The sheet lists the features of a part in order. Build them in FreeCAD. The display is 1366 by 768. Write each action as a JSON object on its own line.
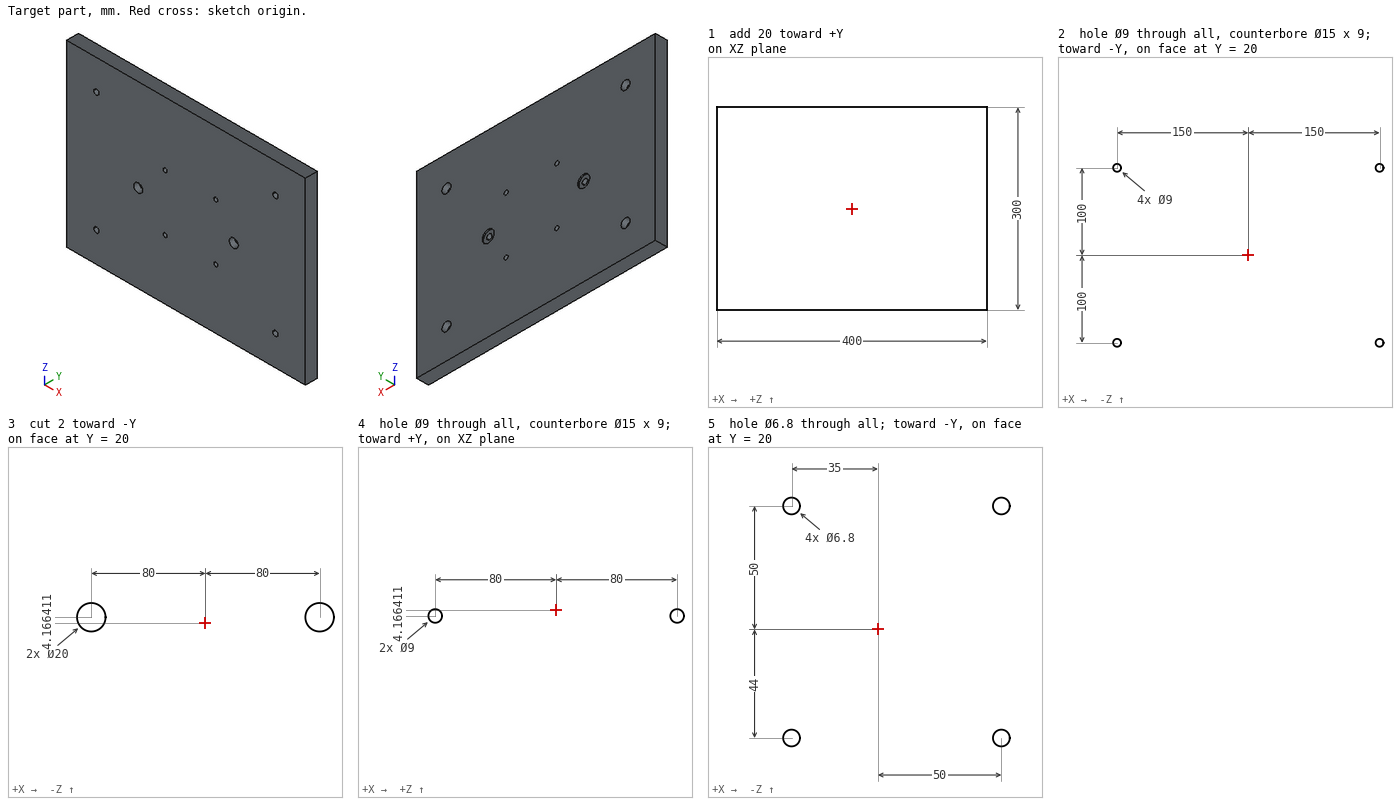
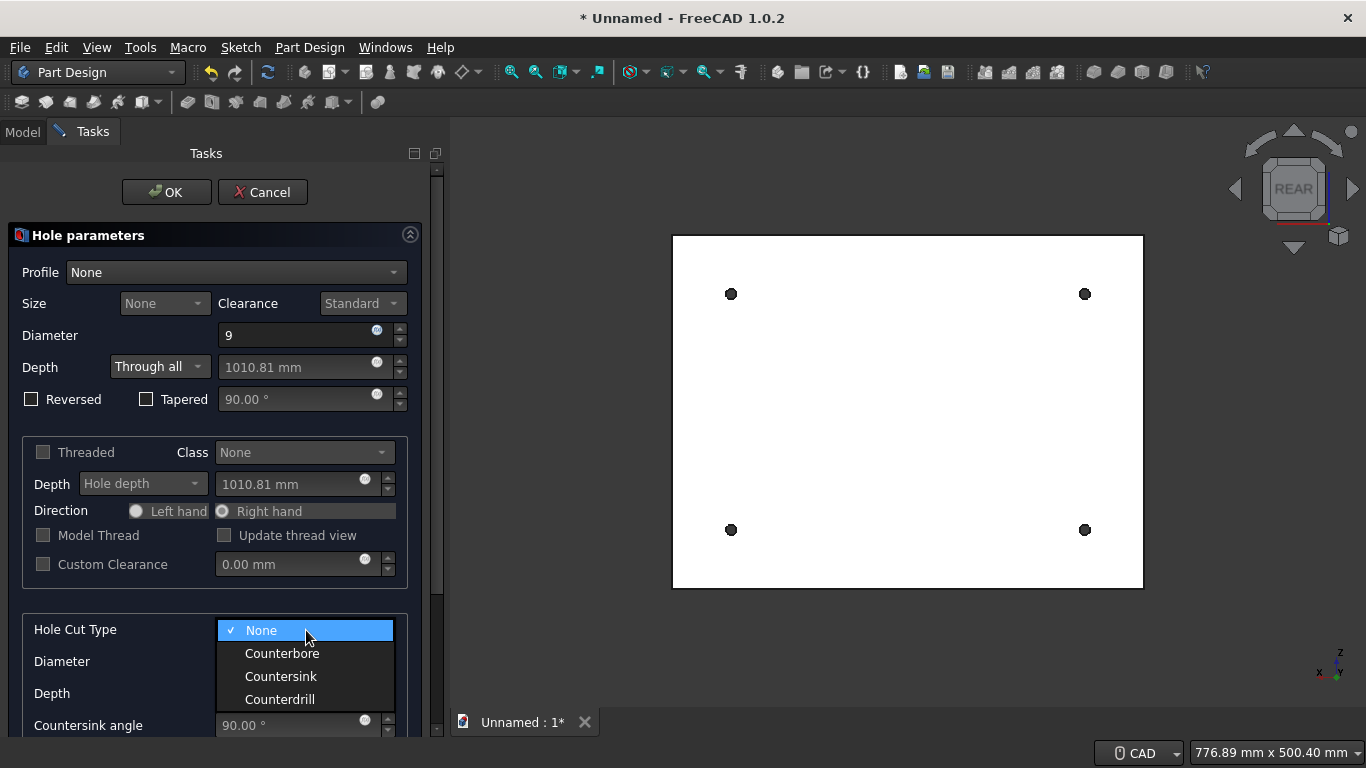
{"action": "left_click", "coordinate": [304, 654]}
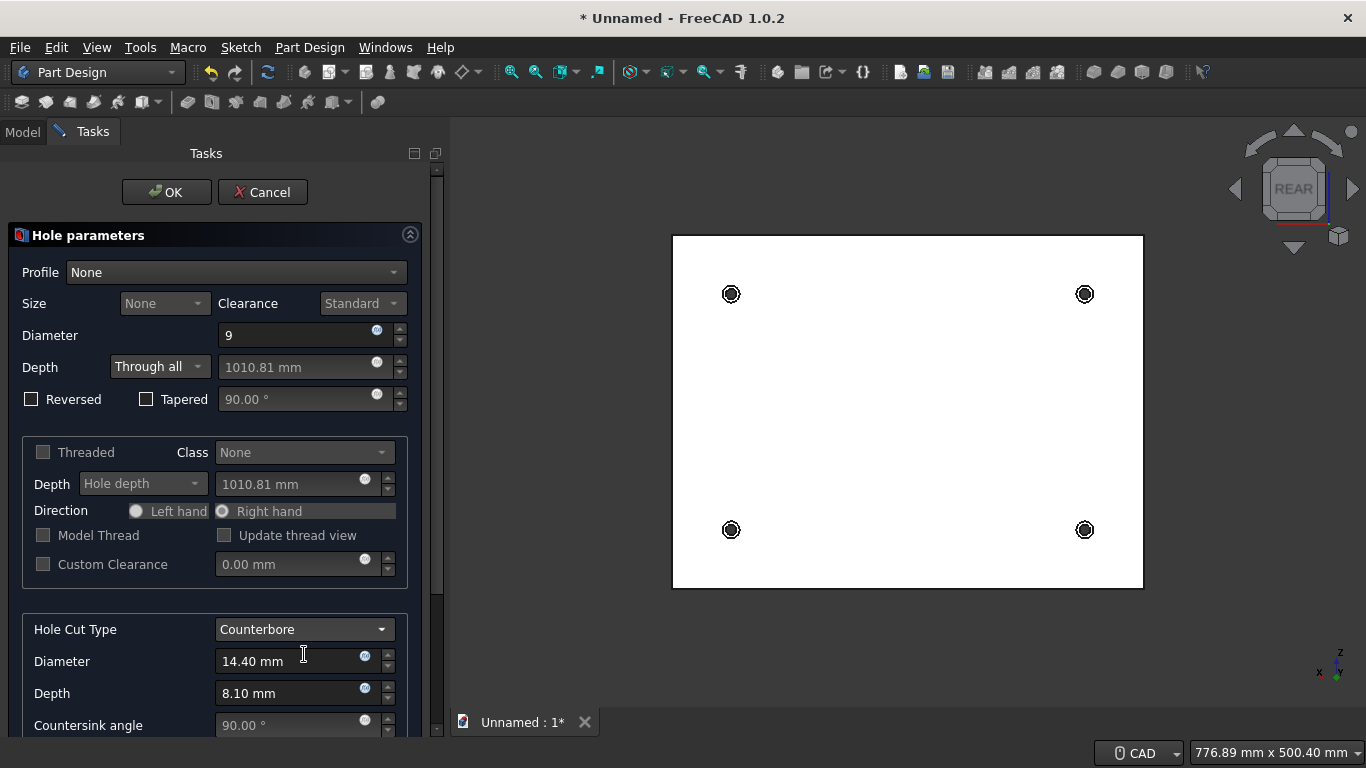
{"action": "triple_click", "coordinate": [298, 661]}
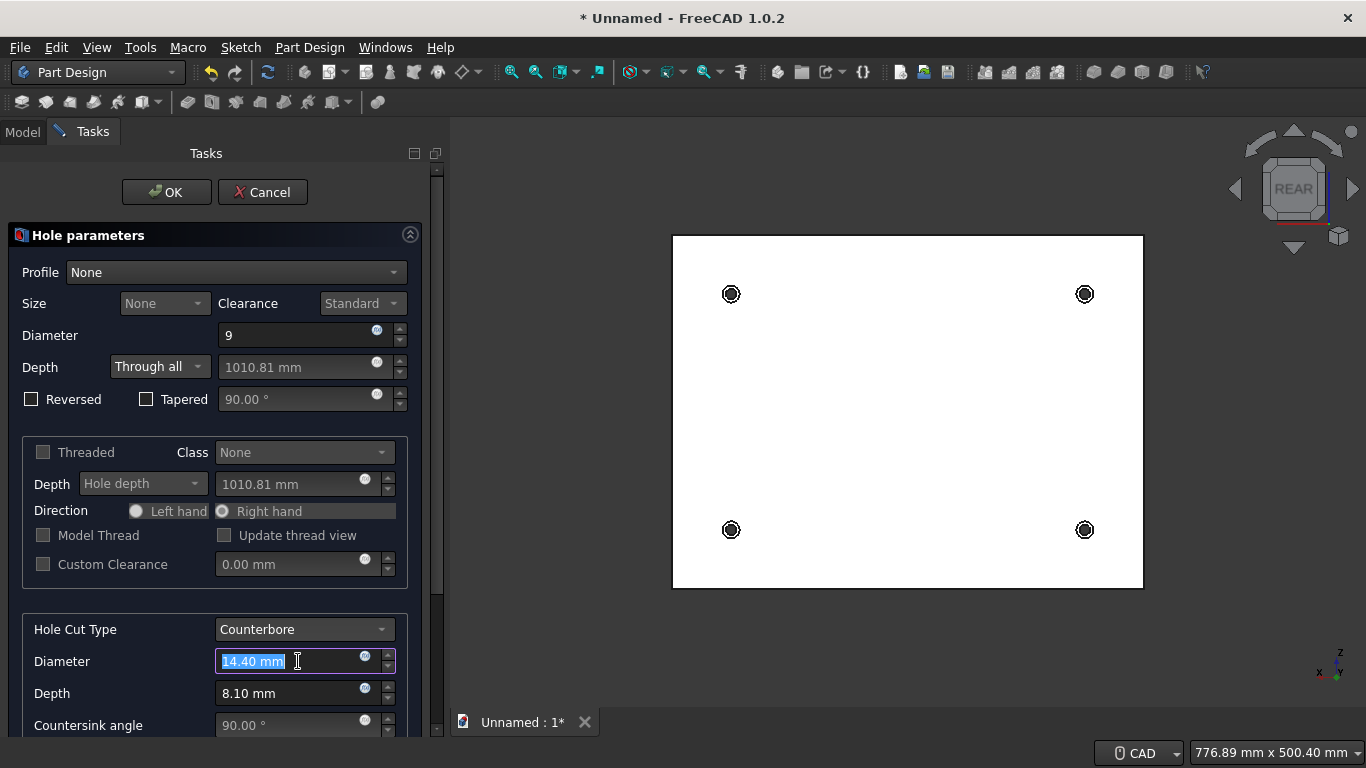
{"action": "type", "text": "15"}
{"action": "key", "text": "Tab"}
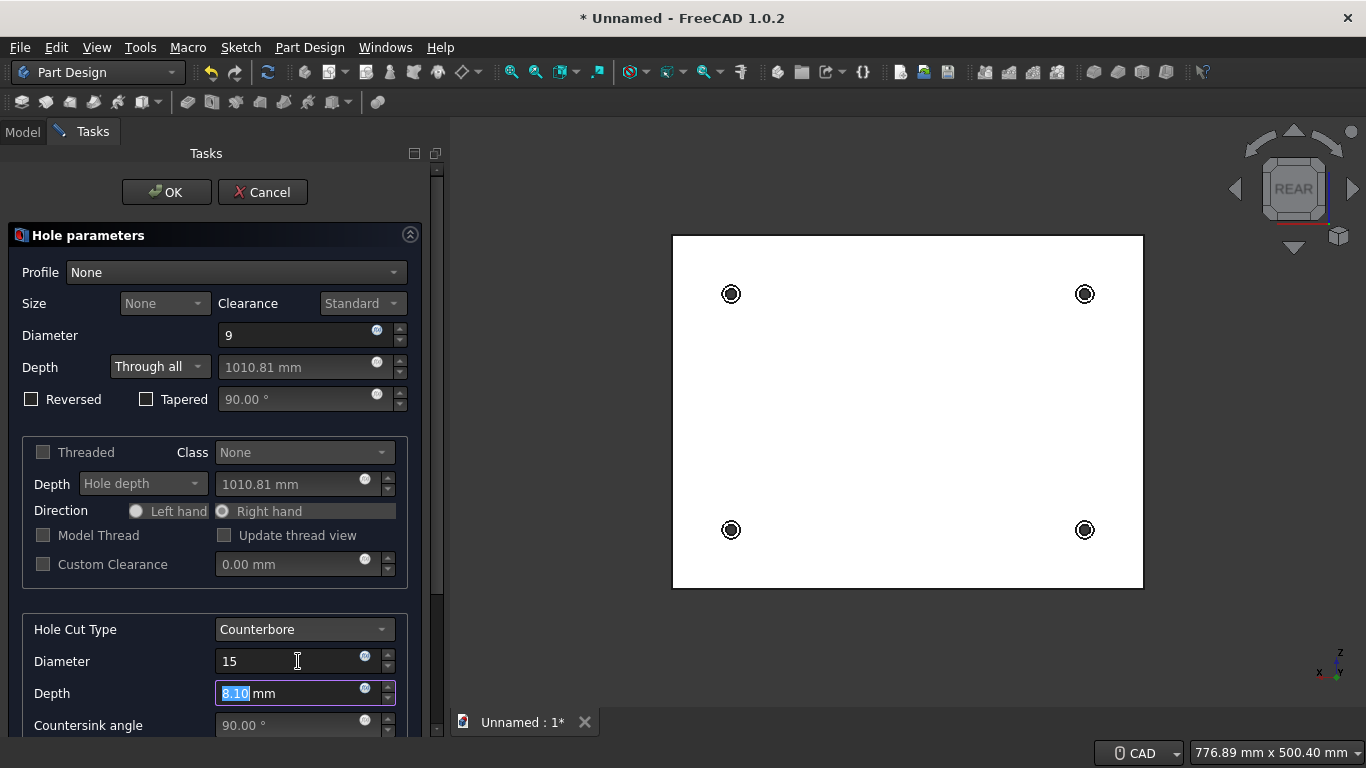
{"action": "type", "text": "9"}
{"action": "key", "text": "Tab"}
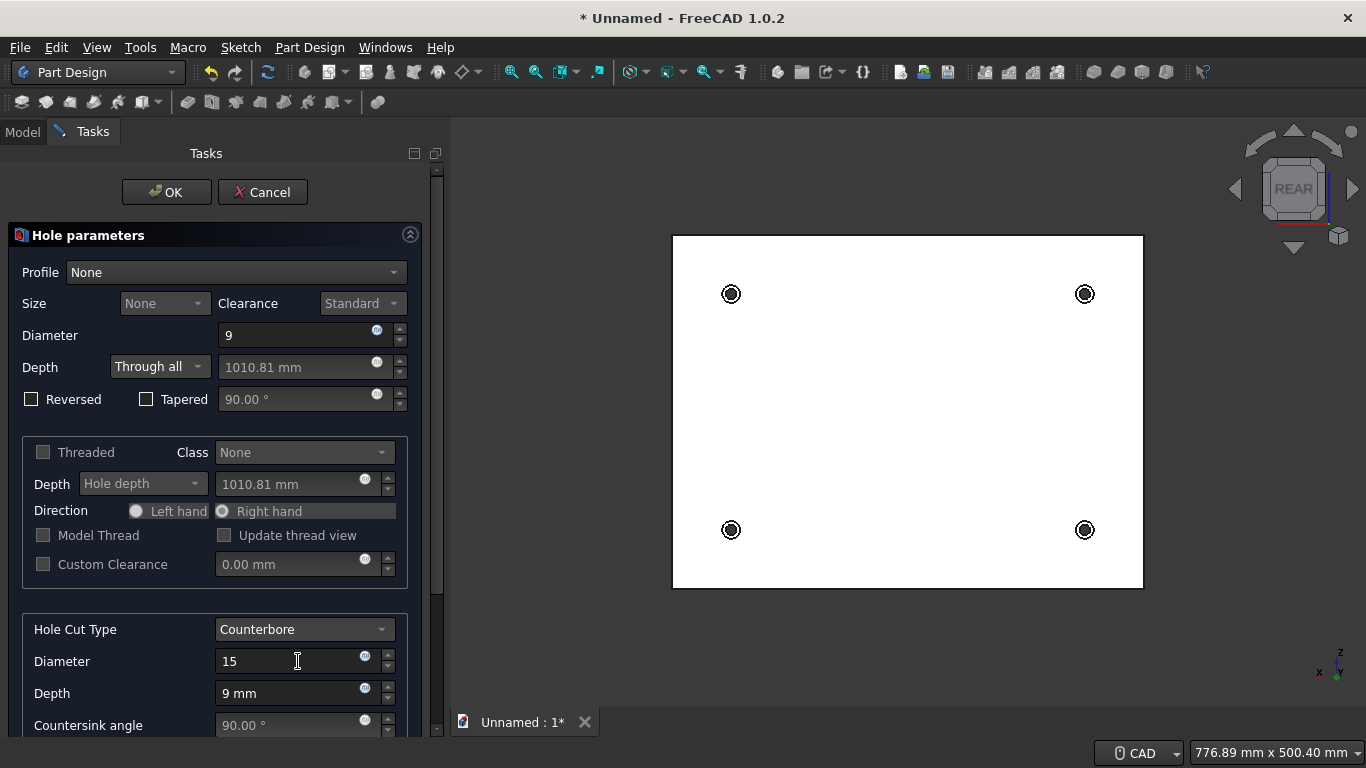
{"action": "left_click", "coordinate": [167, 192]}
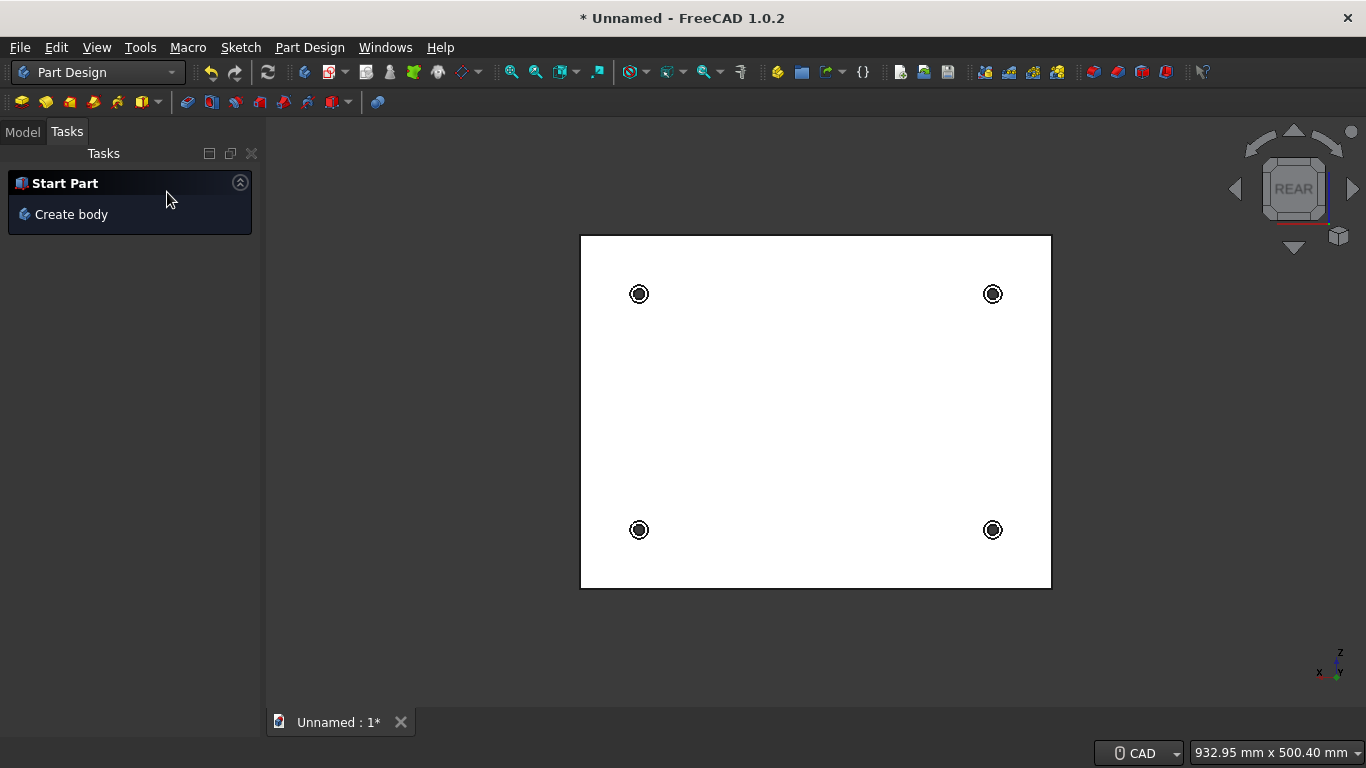
{"action": "left_click", "coordinate": [816, 411]}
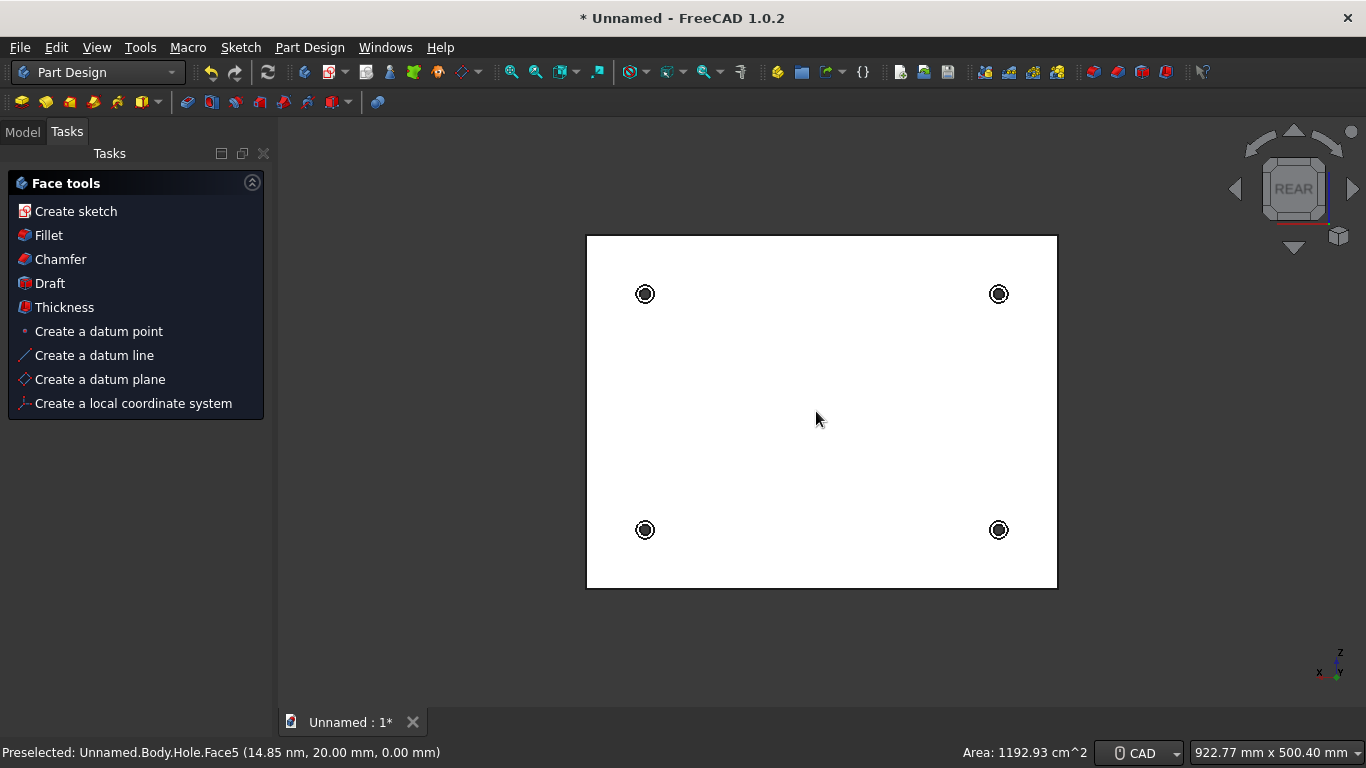
{"action": "left_click", "coordinate": [330, 72]}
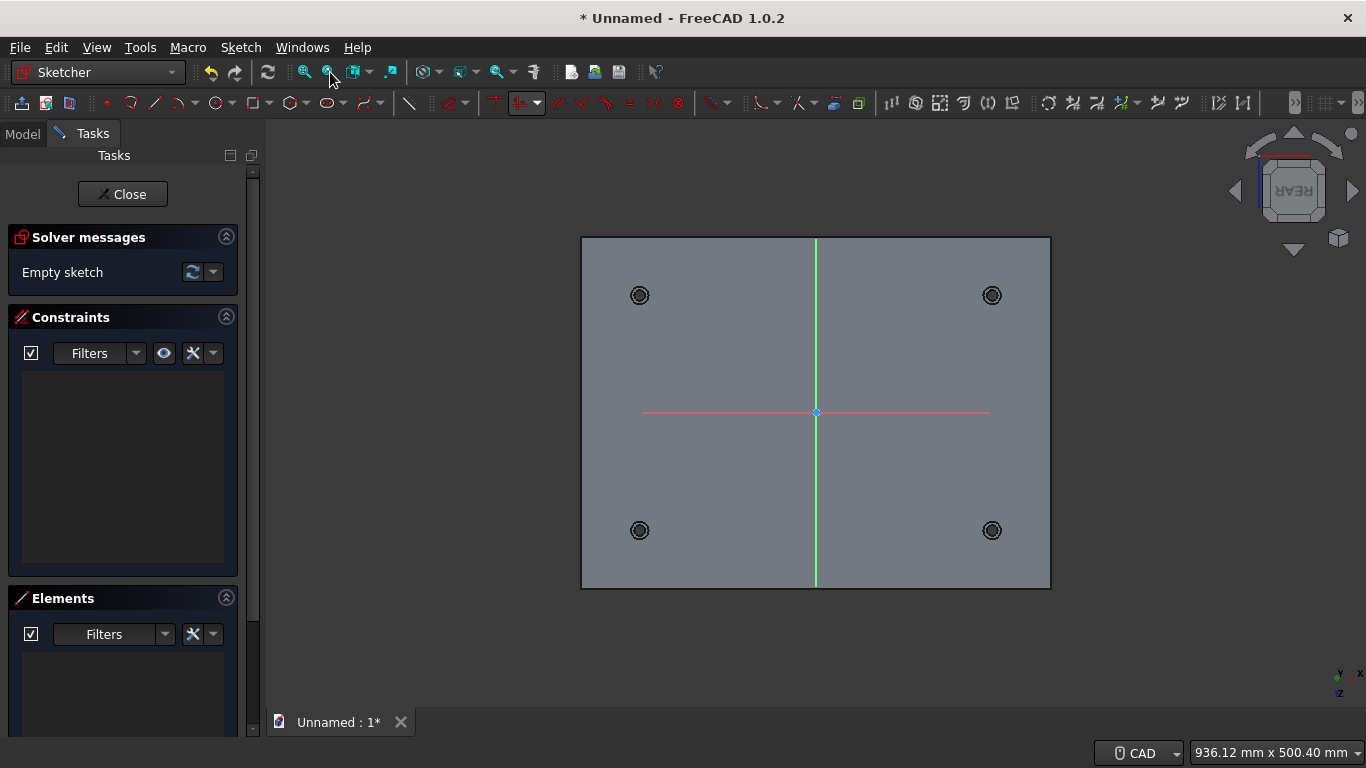
{"action": "scroll", "coordinate": [846, 406], "scroll_direction": "up", "scroll_amount": 6}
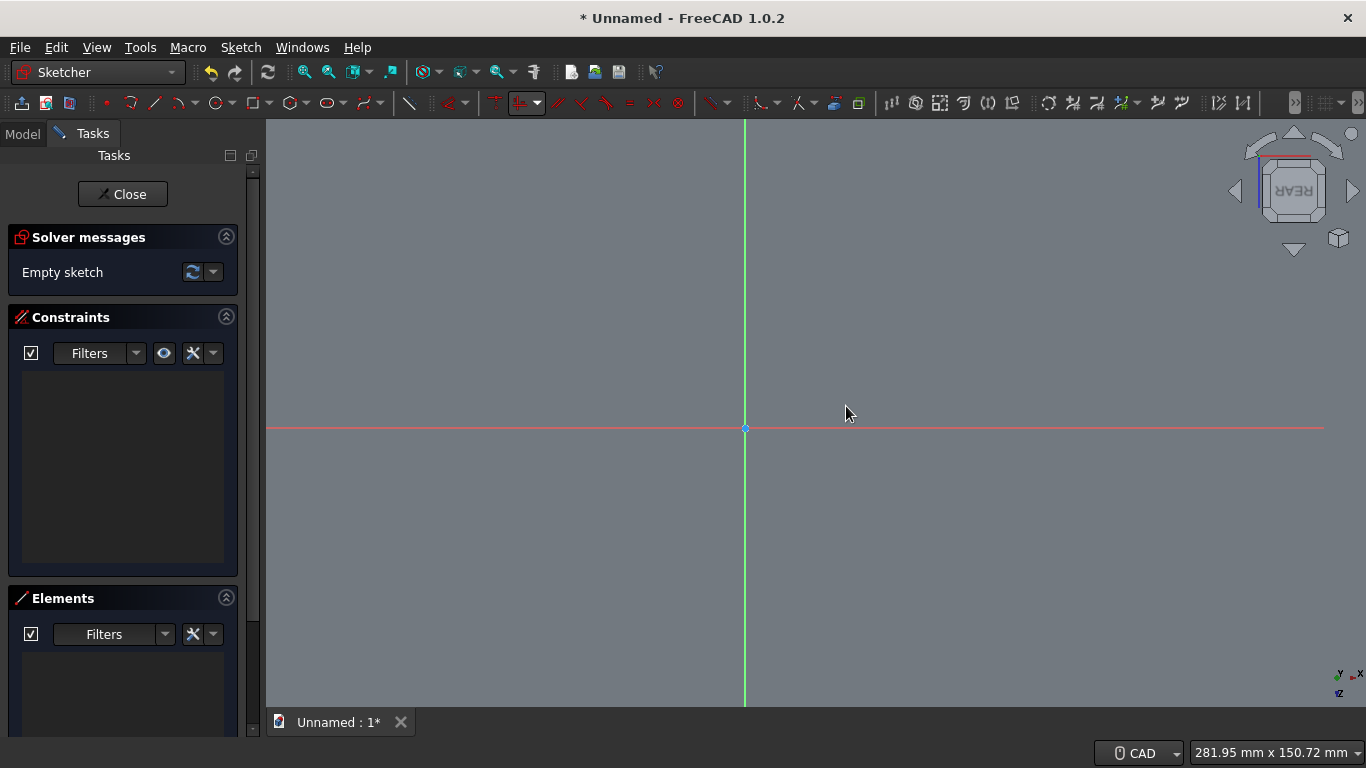
{"action": "left_click", "coordinate": [216, 104]}